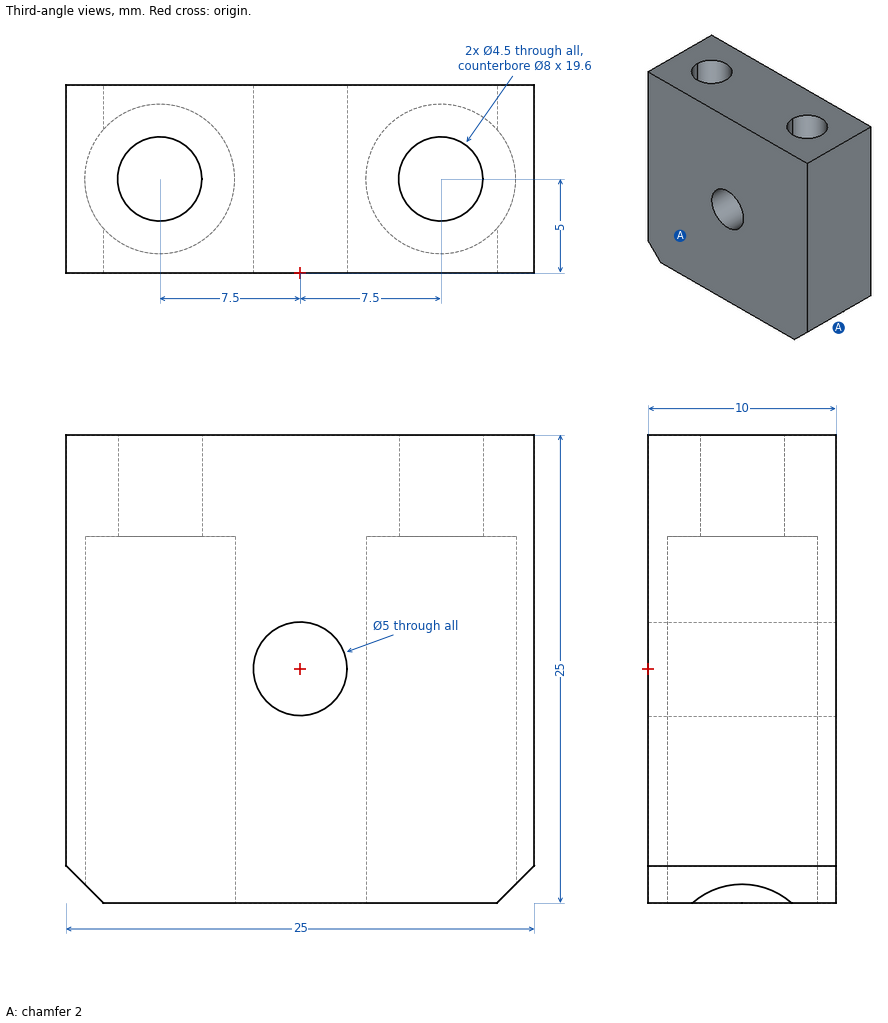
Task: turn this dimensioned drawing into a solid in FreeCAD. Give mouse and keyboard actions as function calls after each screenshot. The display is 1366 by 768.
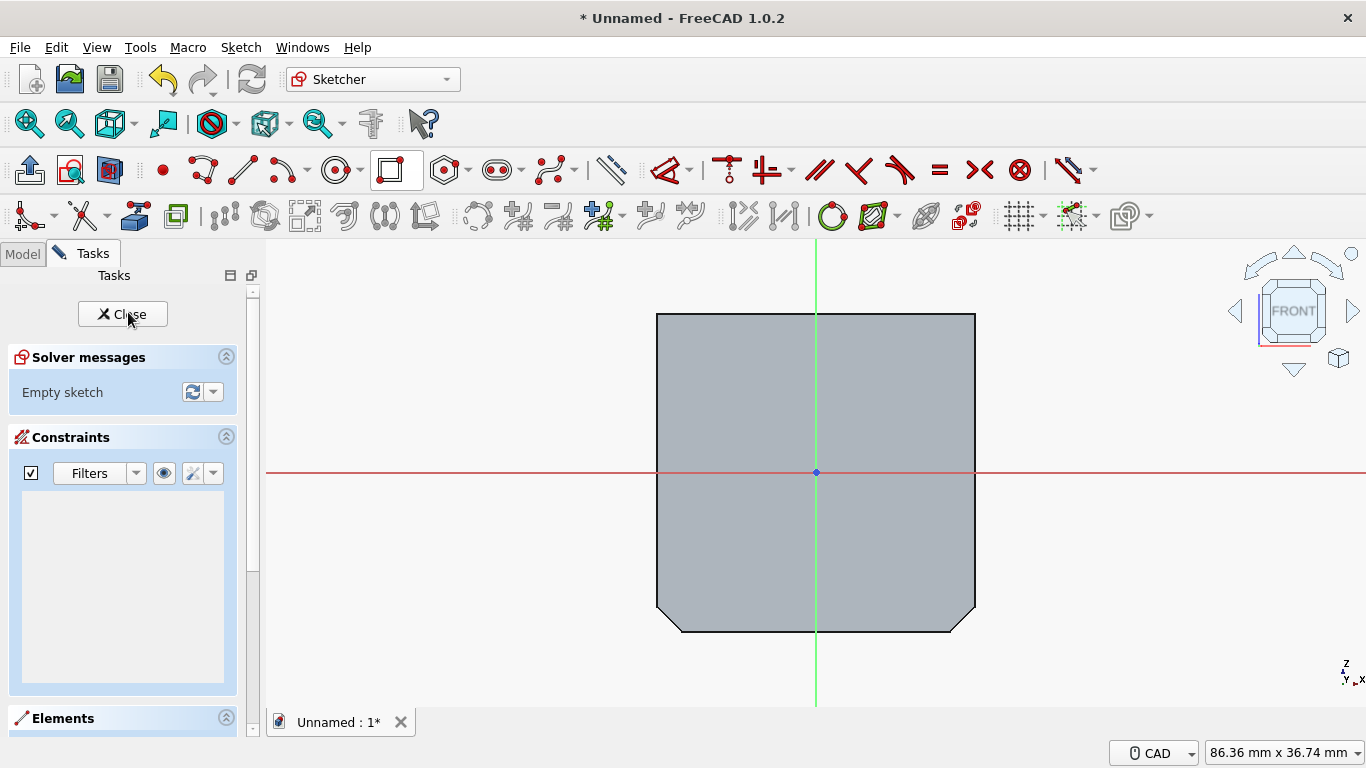
scroll(833, 473, up, 8)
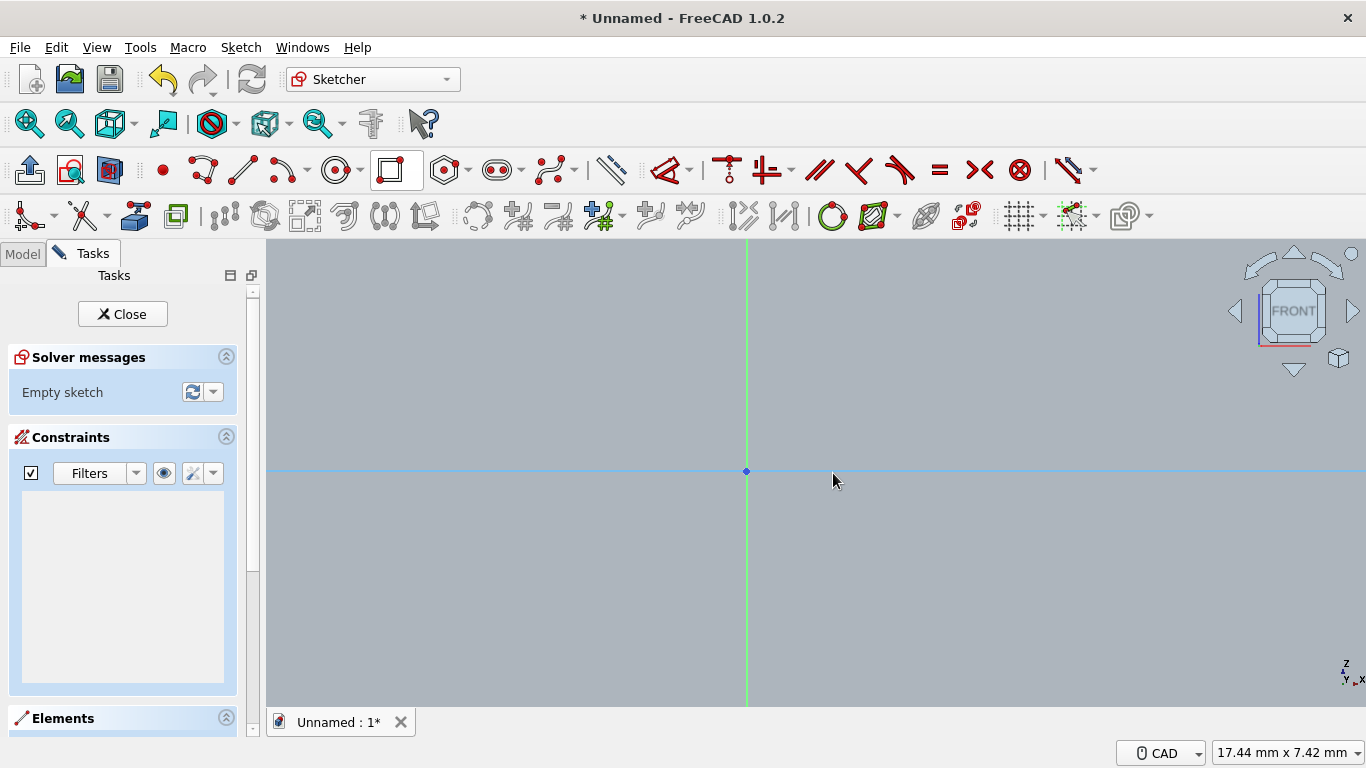
key(g)
key(c)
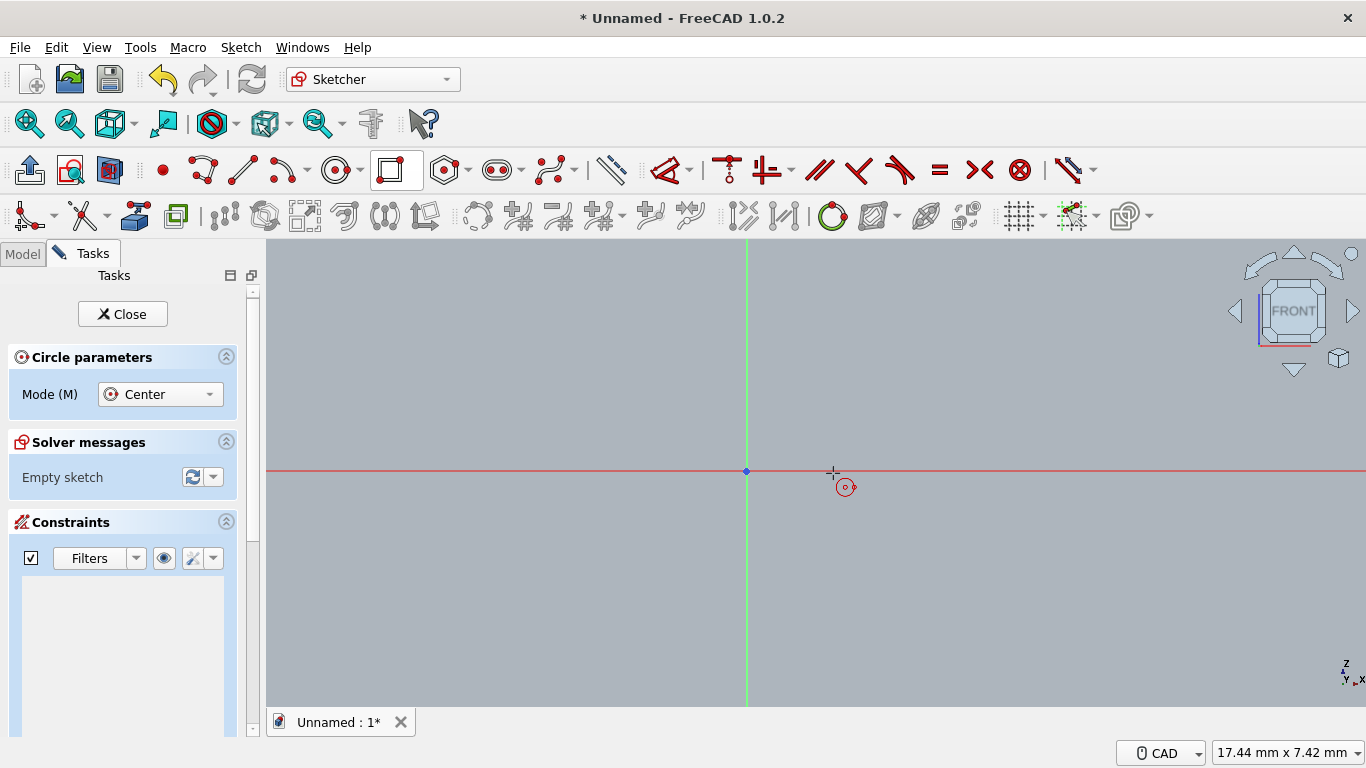
click(747, 471)
move(858, 359)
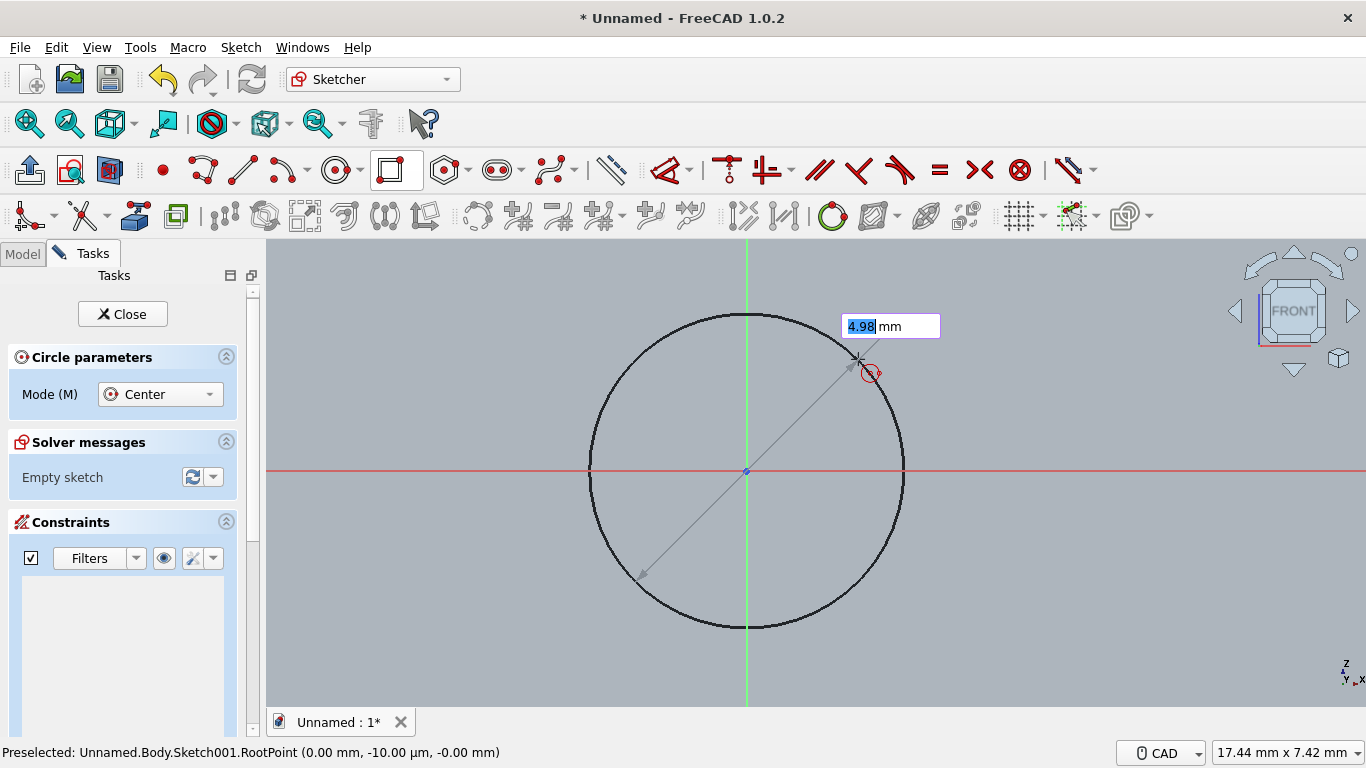
text(5)
key(Return)
key(Escape)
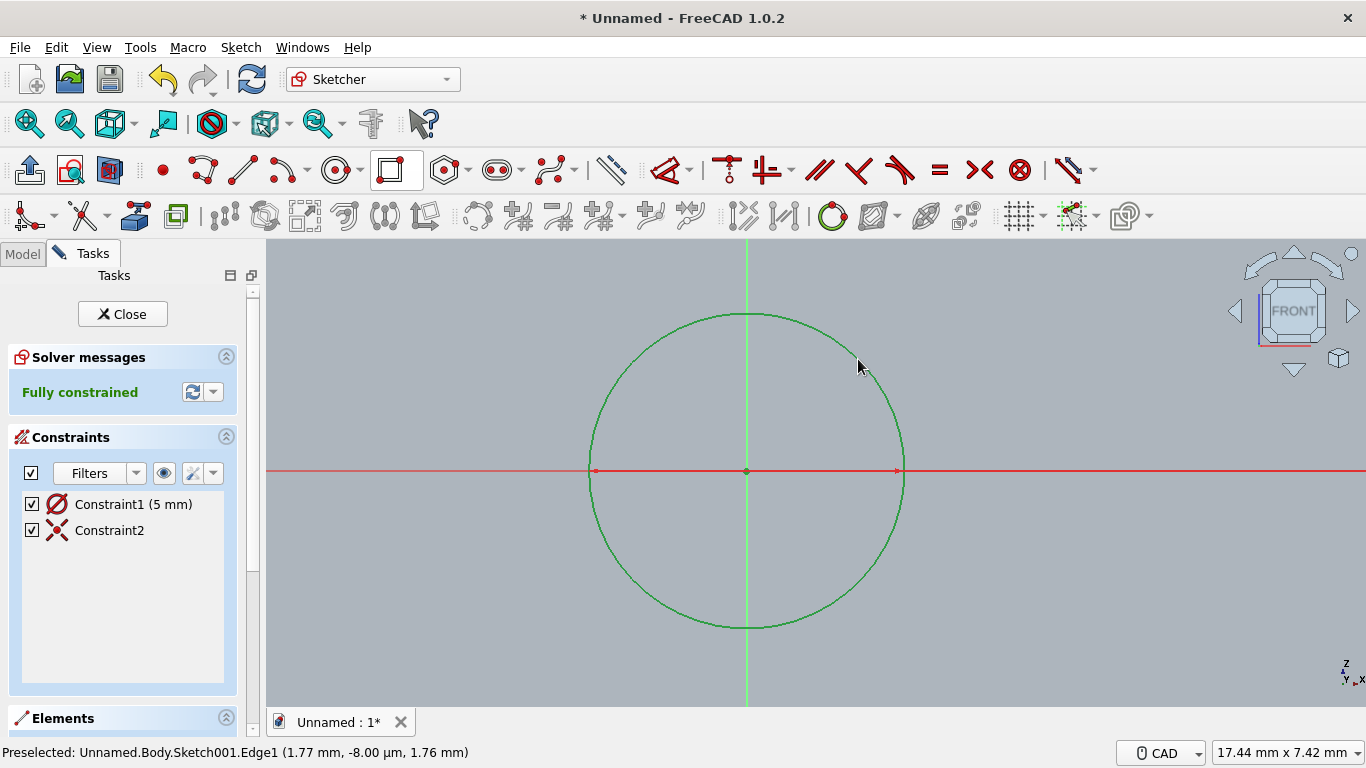
click(123, 314)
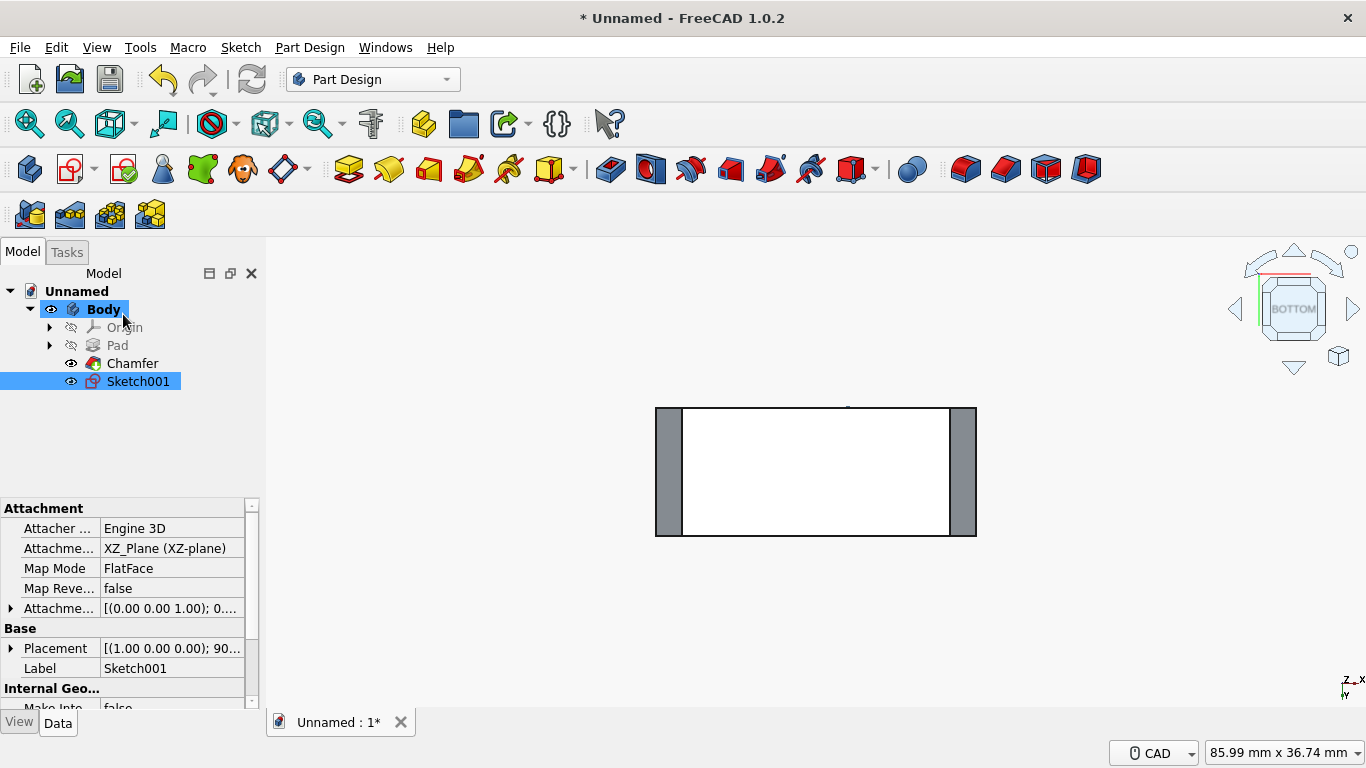
click(652, 170)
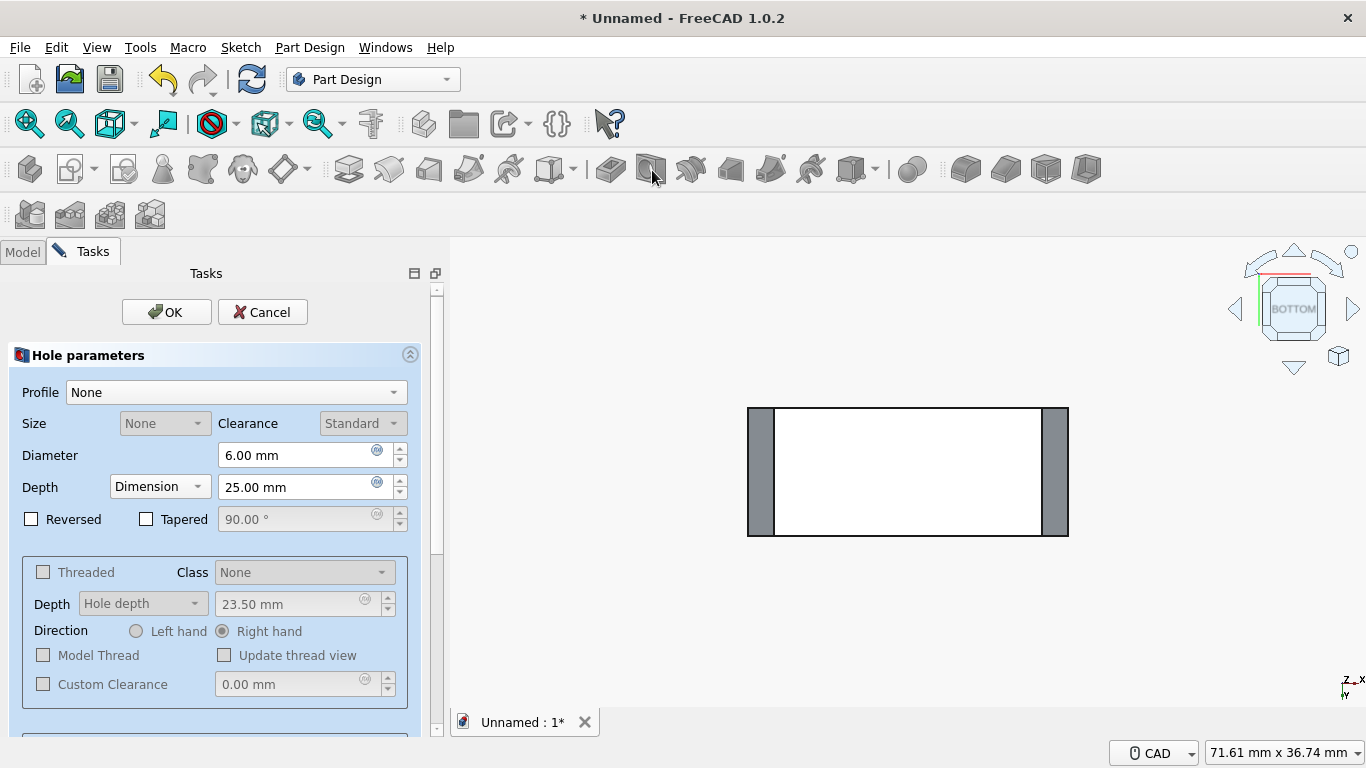
triple_click(305, 455)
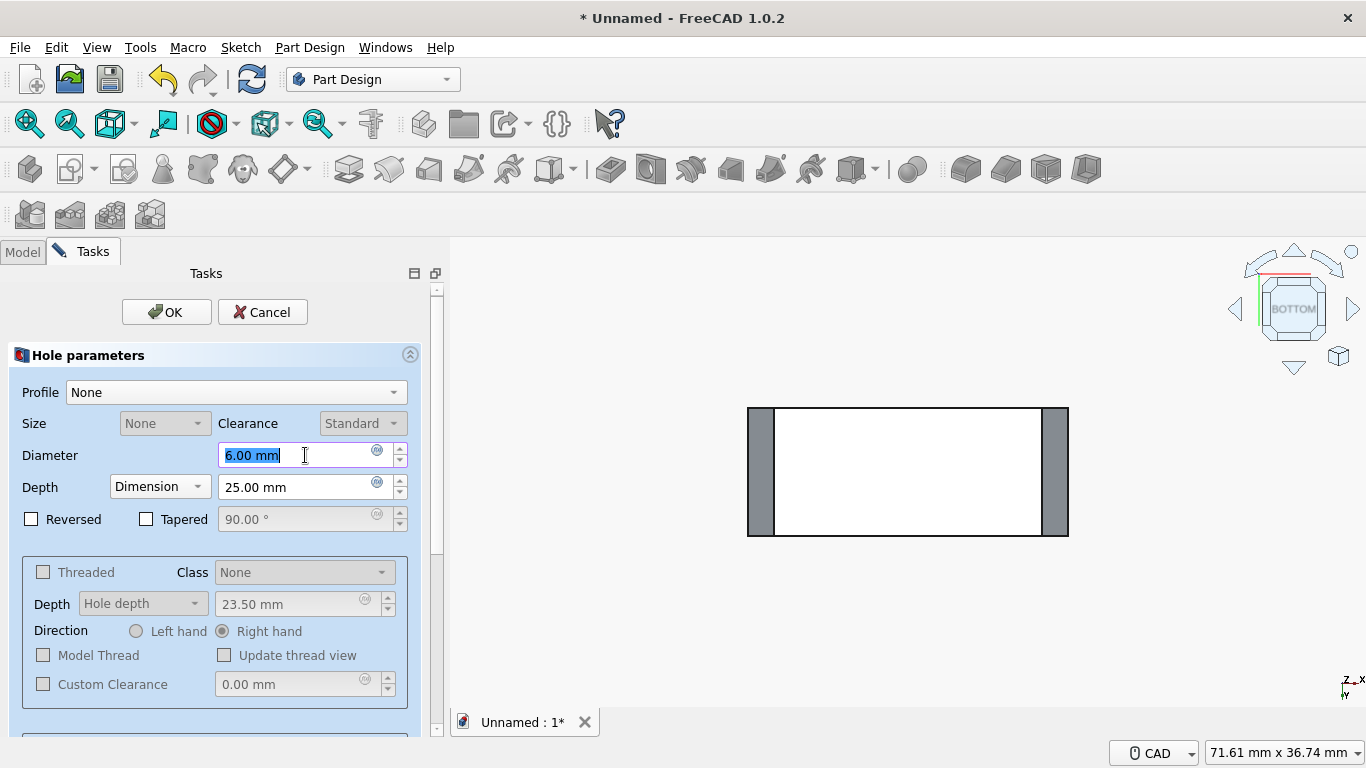
text(5)
key(Tab)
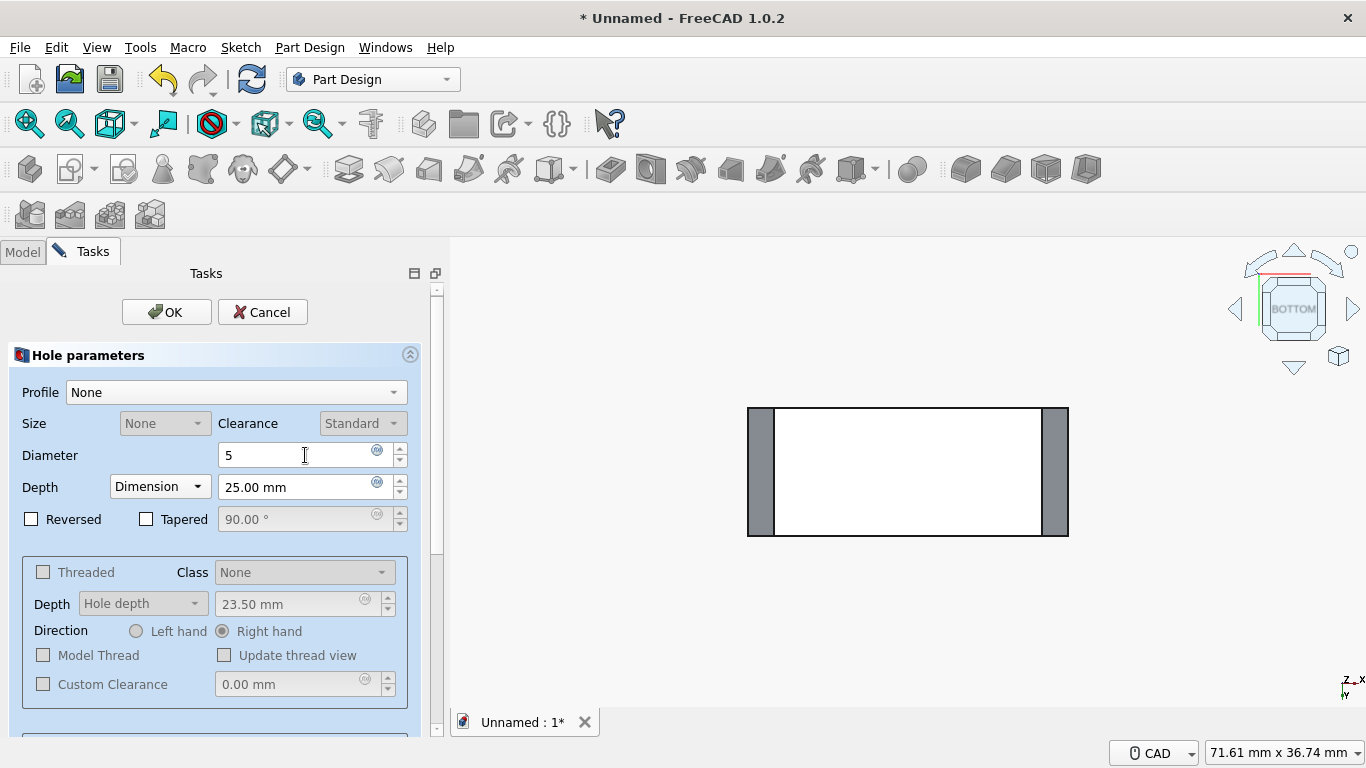
click(161, 486)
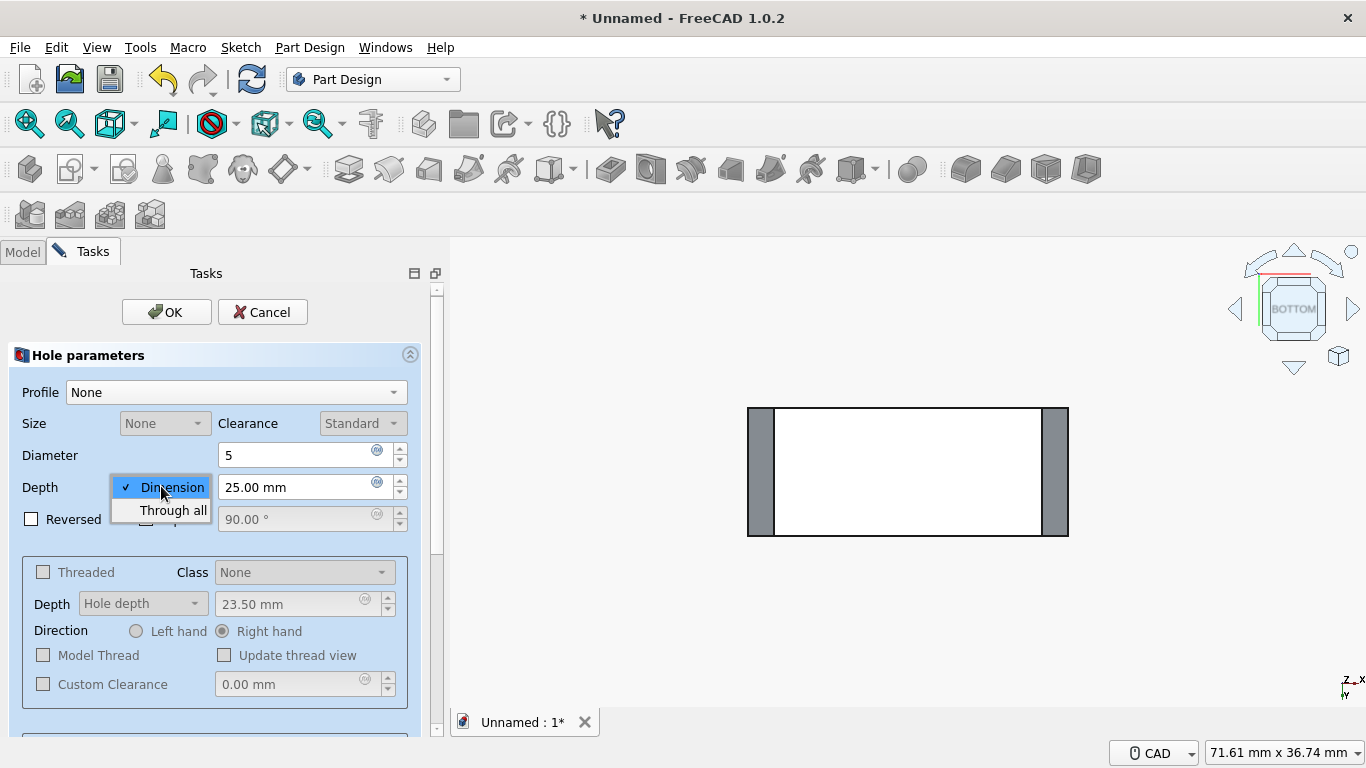
click(160, 510)